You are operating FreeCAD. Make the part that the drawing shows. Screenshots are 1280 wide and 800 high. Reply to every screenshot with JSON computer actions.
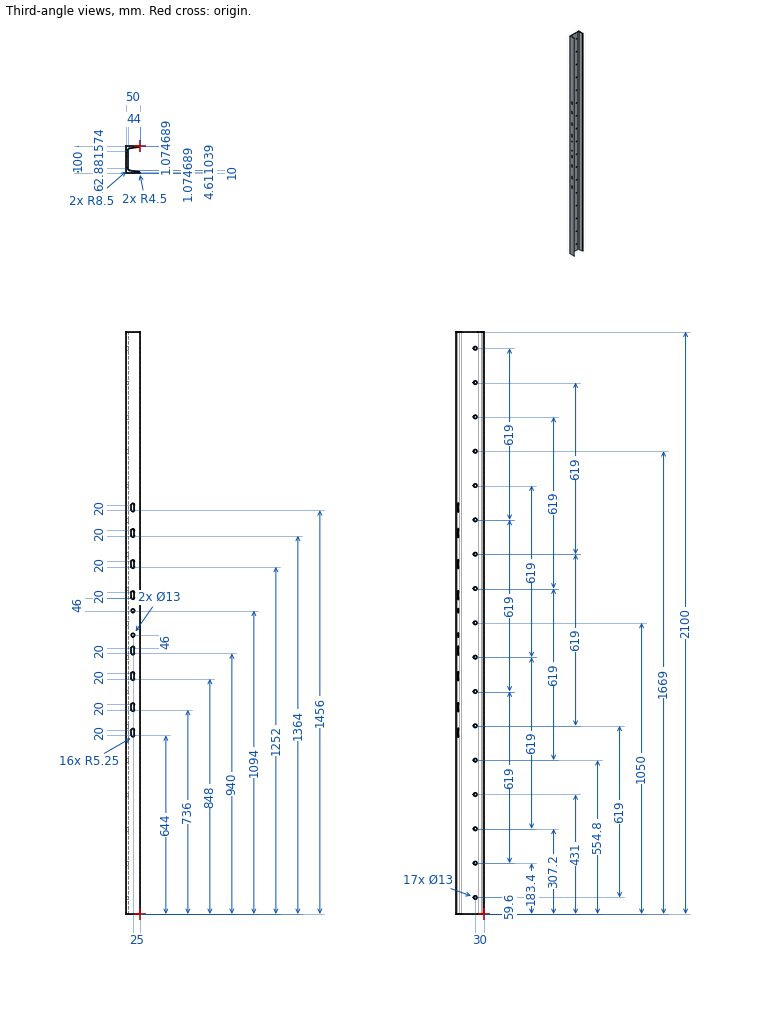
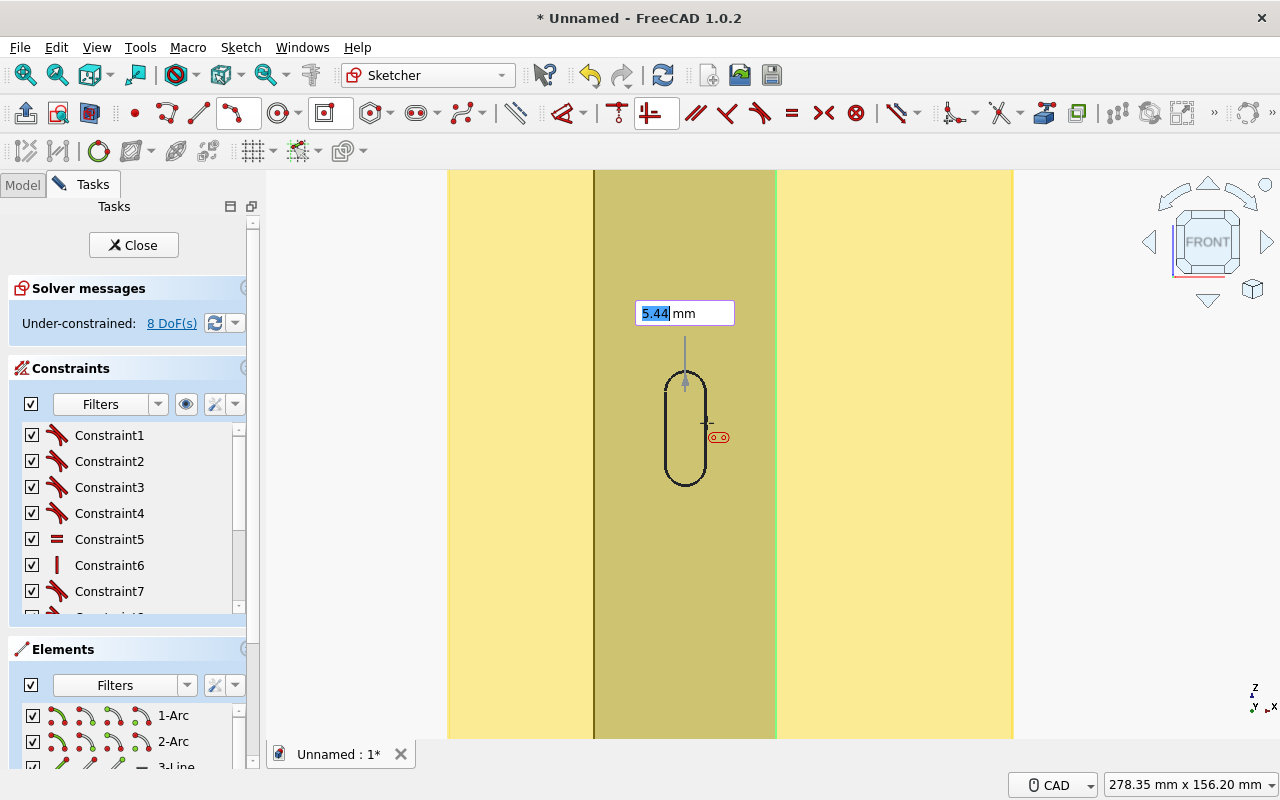
{"action": "left_click", "coordinate": [704, 422]}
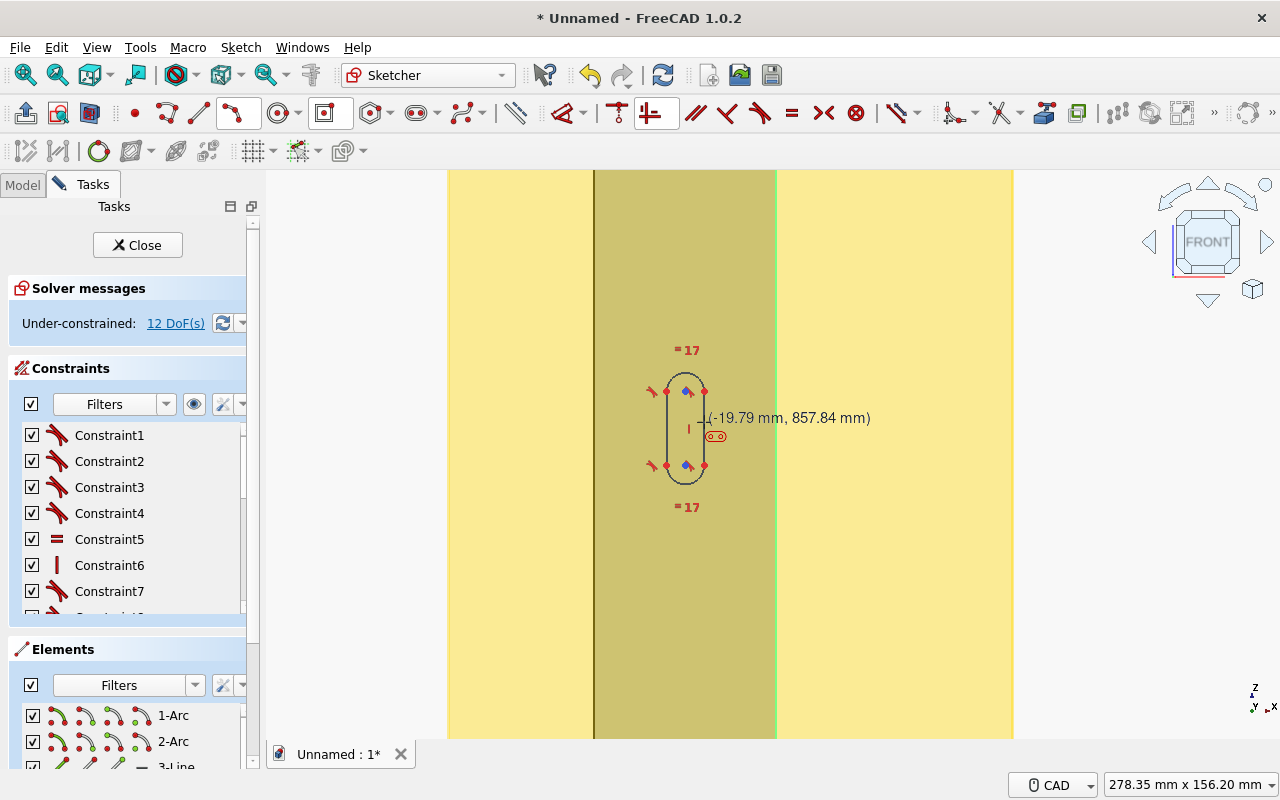
{"action": "scroll", "coordinate": [704, 429], "scroll_direction": "down", "scroll_amount": 14}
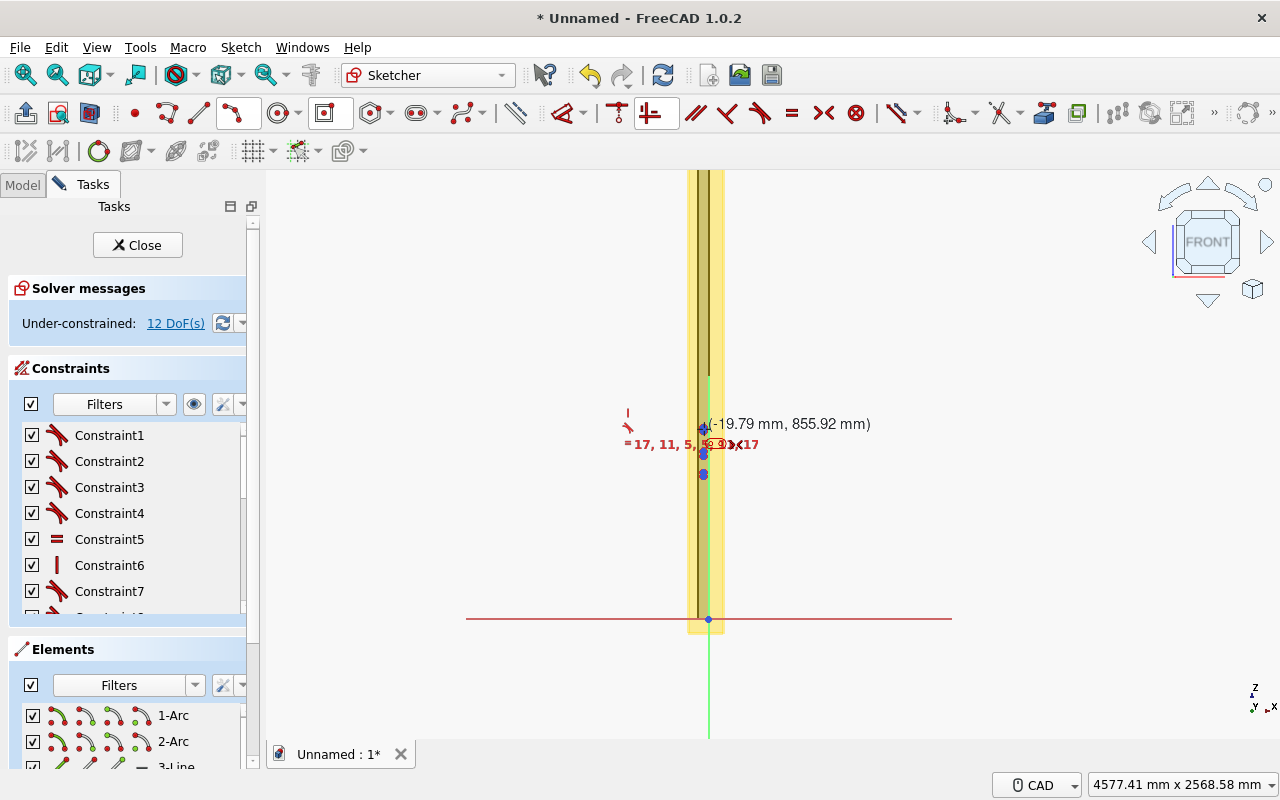
{"action": "scroll", "coordinate": [703, 411], "scroll_direction": "up", "scroll_amount": 15}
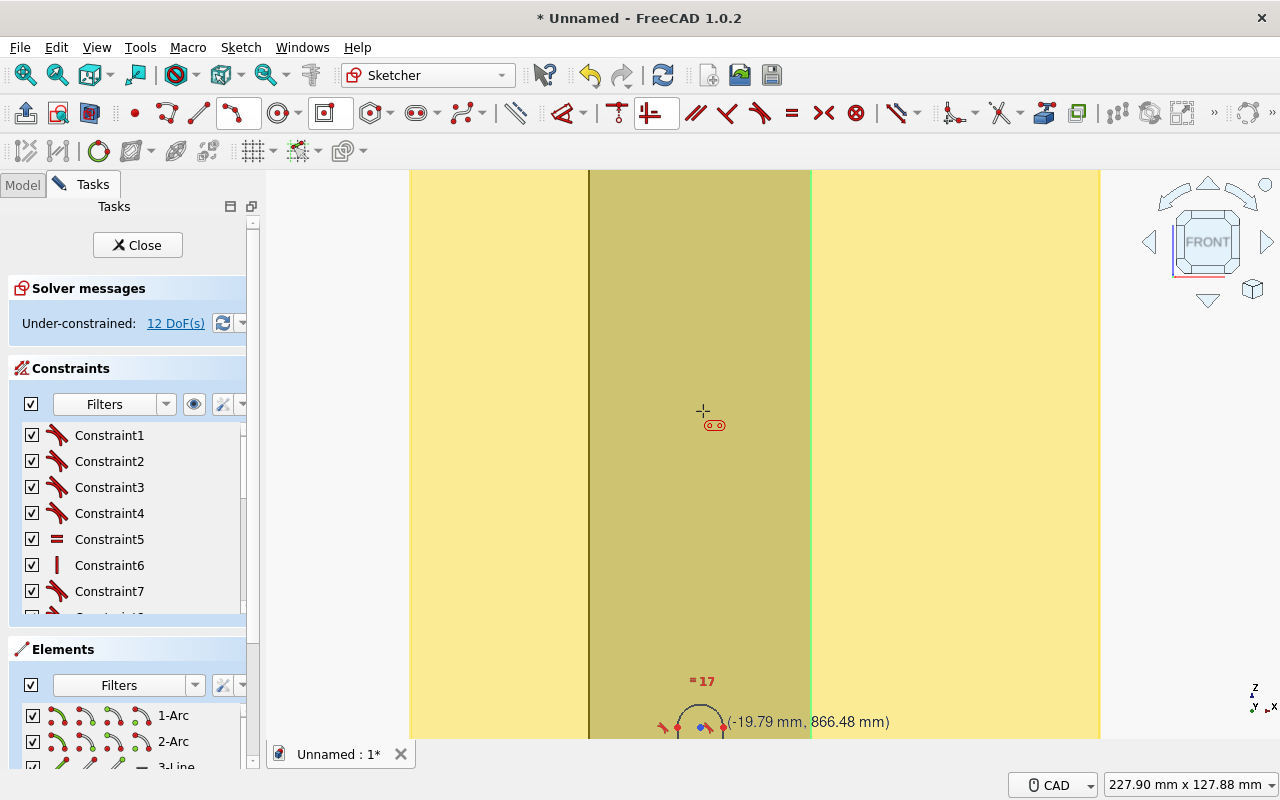
{"action": "scroll", "coordinate": [703, 411], "scroll_direction": "down", "scroll_amount": 15}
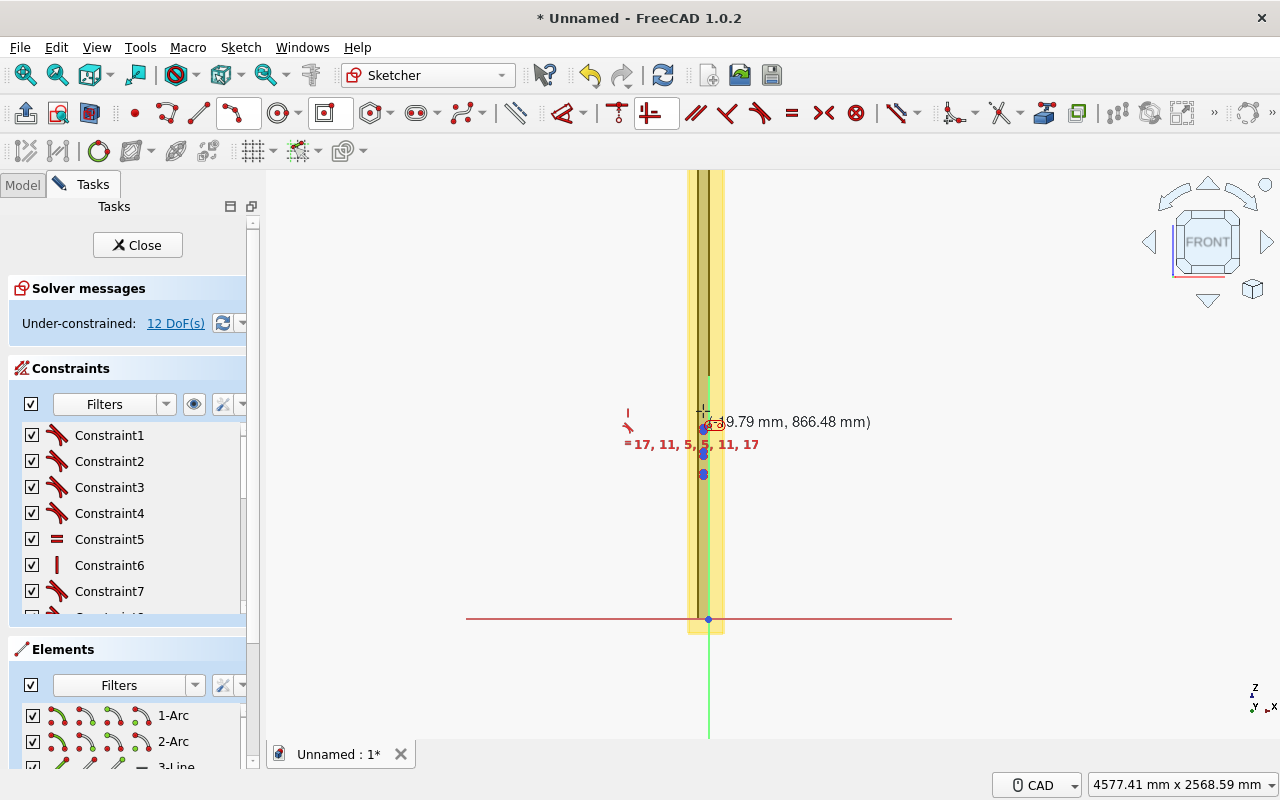
{"action": "scroll", "coordinate": [703, 411], "scroll_direction": "up", "scroll_amount": 6}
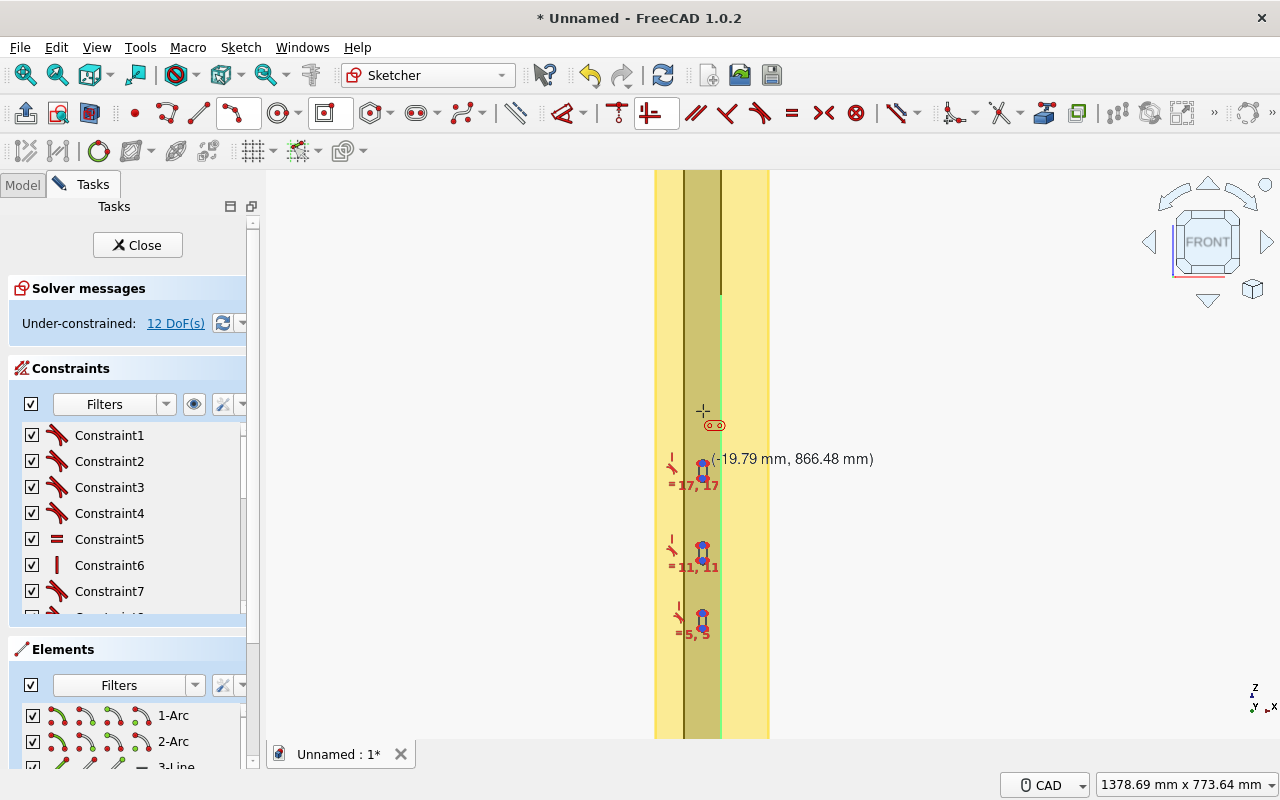
{"action": "left_click", "coordinate": [703, 410]}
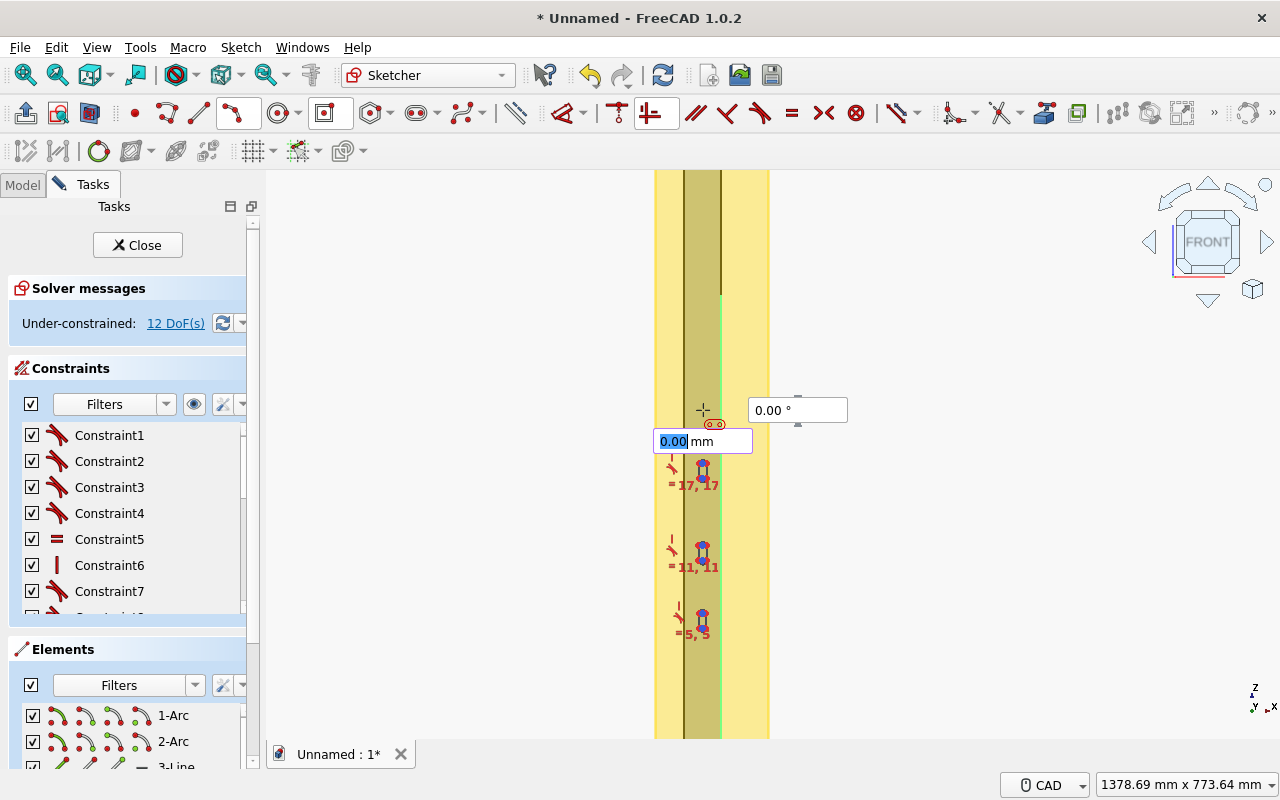
{"action": "left_click", "coordinate": [703, 395]}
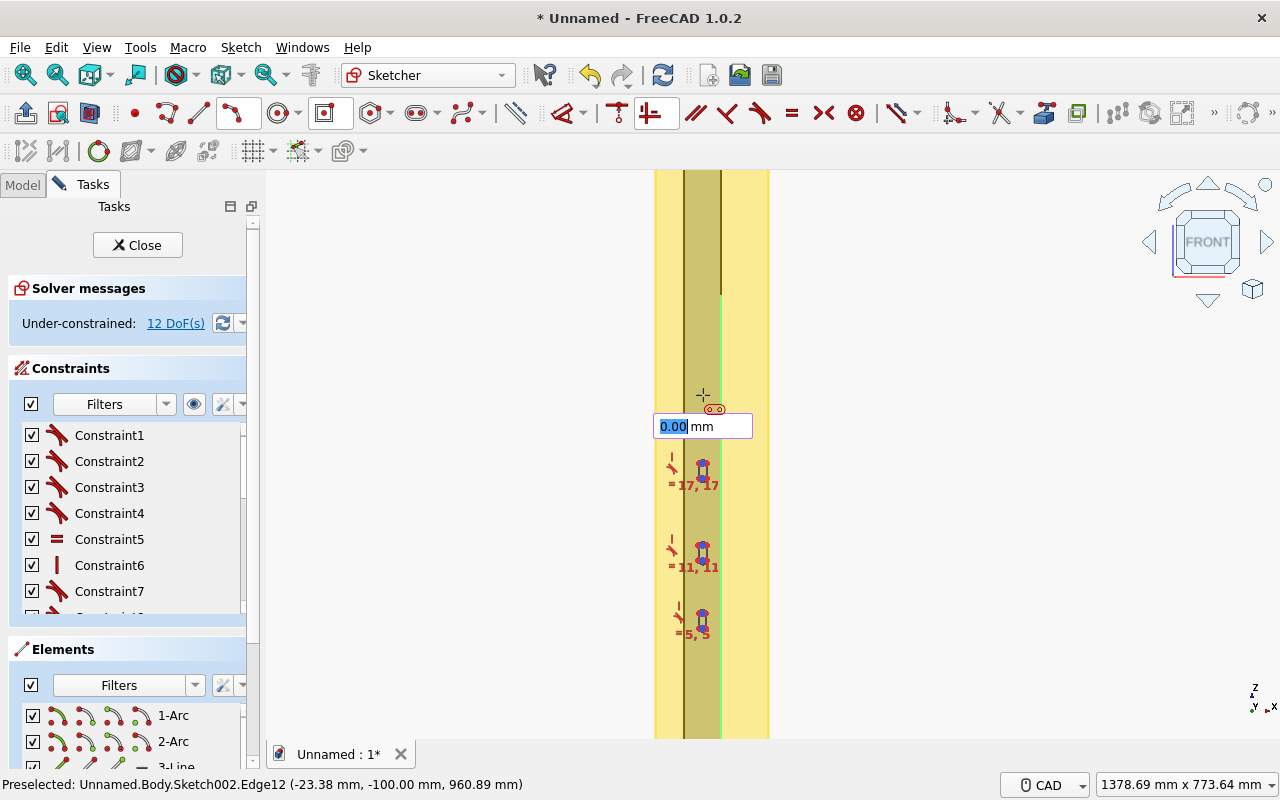
{"action": "scroll", "coordinate": [707, 402], "scroll_direction": "up", "scroll_amount": 8}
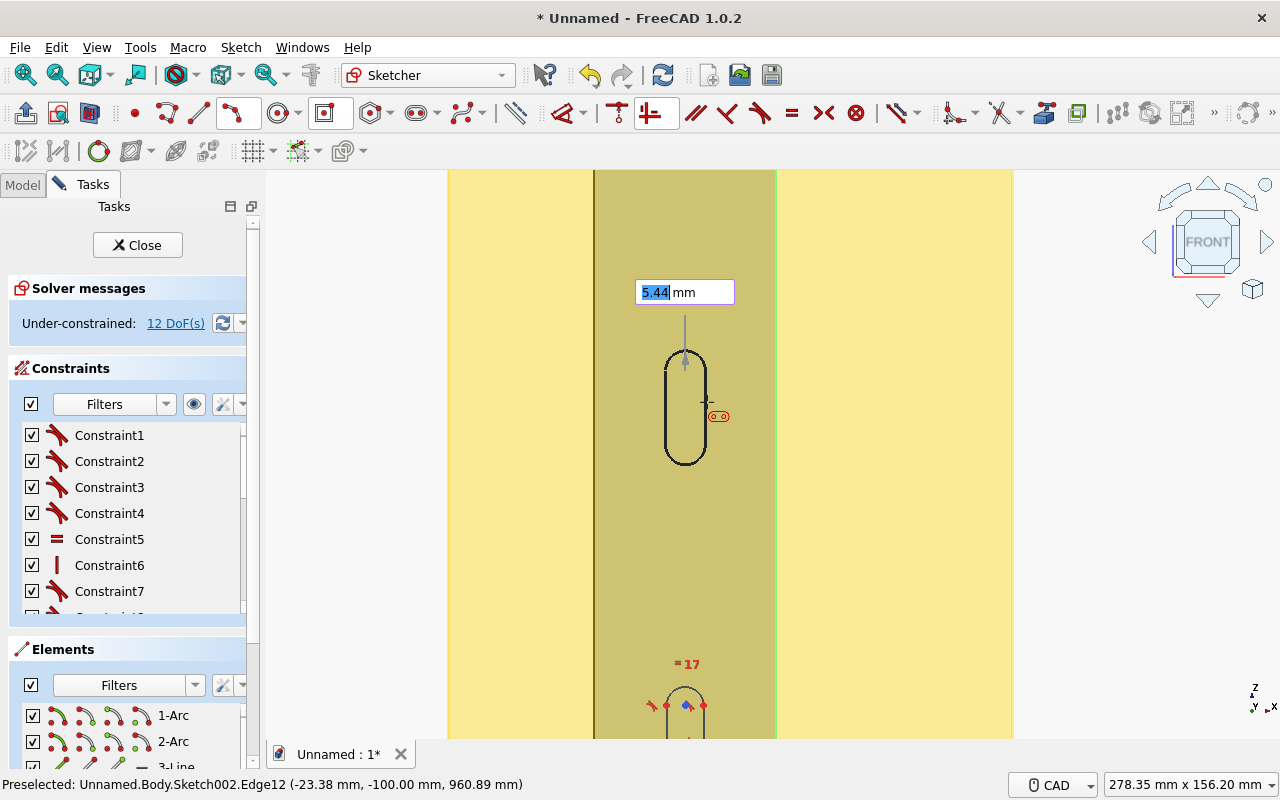
{"action": "left_click", "coordinate": [704, 401]}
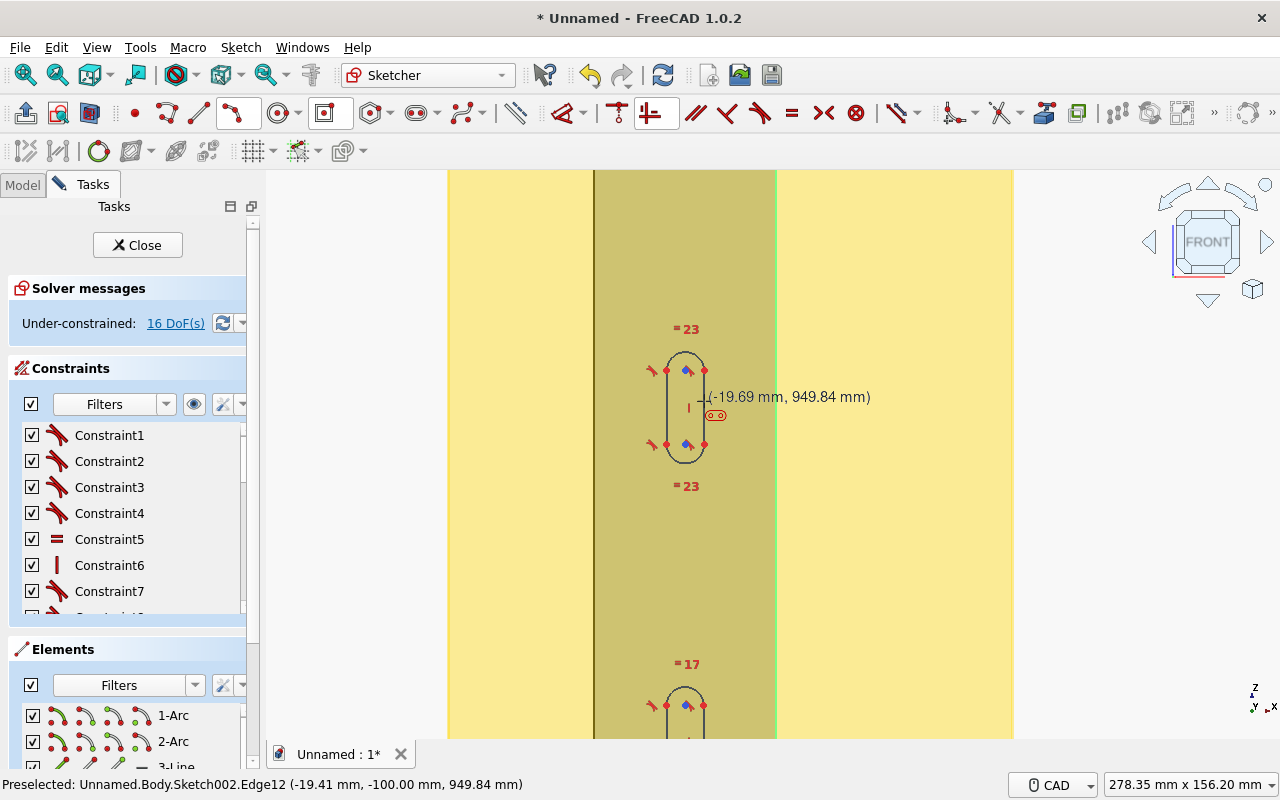
{"action": "scroll", "coordinate": [704, 409], "scroll_direction": "down", "scroll_amount": 14}